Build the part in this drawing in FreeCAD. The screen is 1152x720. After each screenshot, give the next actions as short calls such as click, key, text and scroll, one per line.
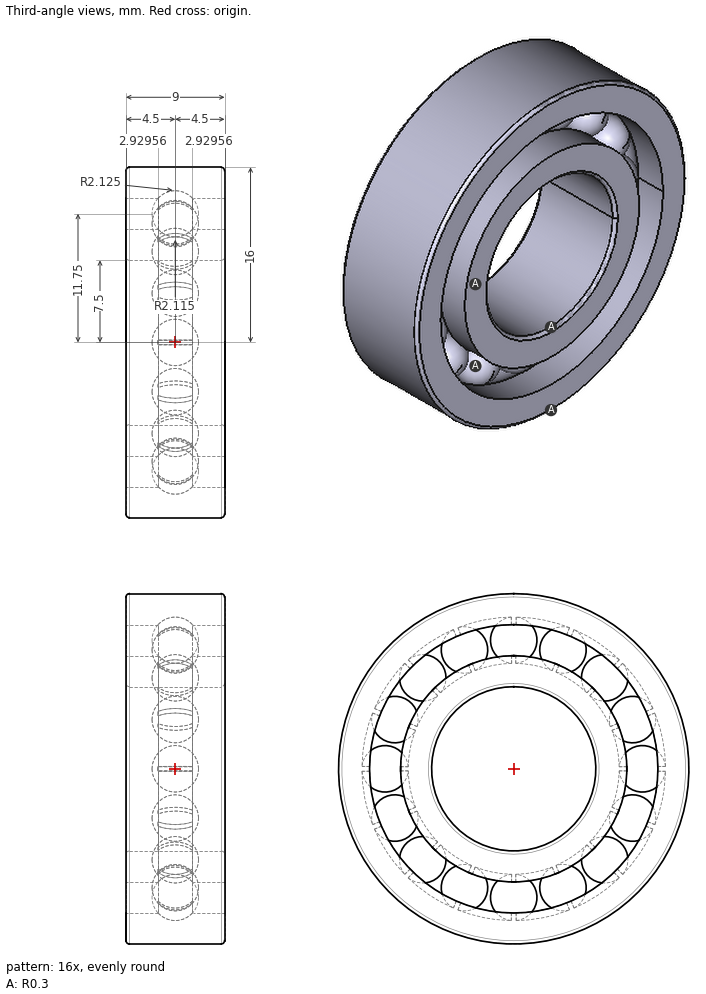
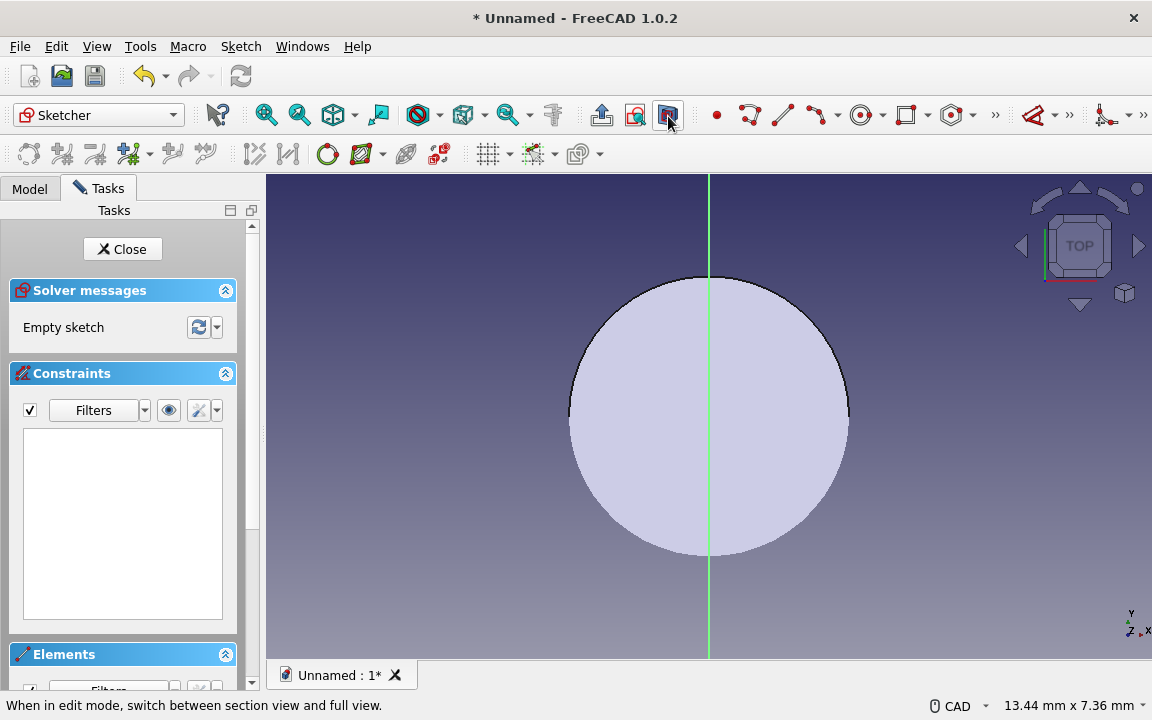
scroll(601, 202, down, 5)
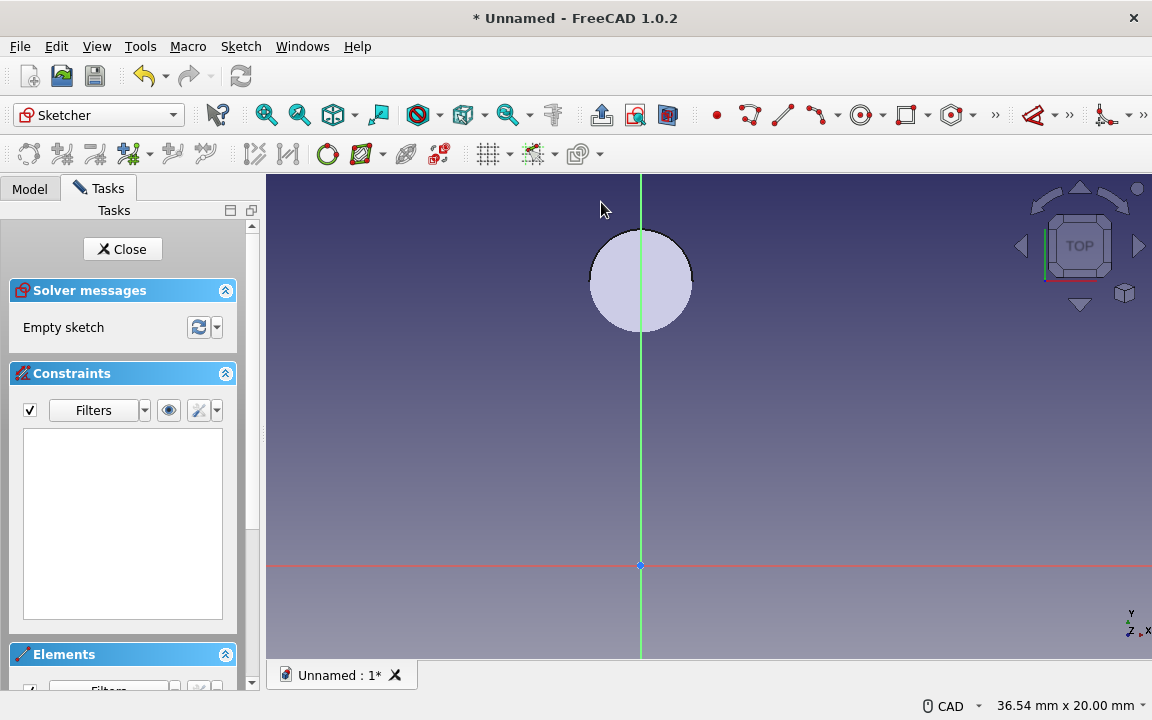
click(750, 116)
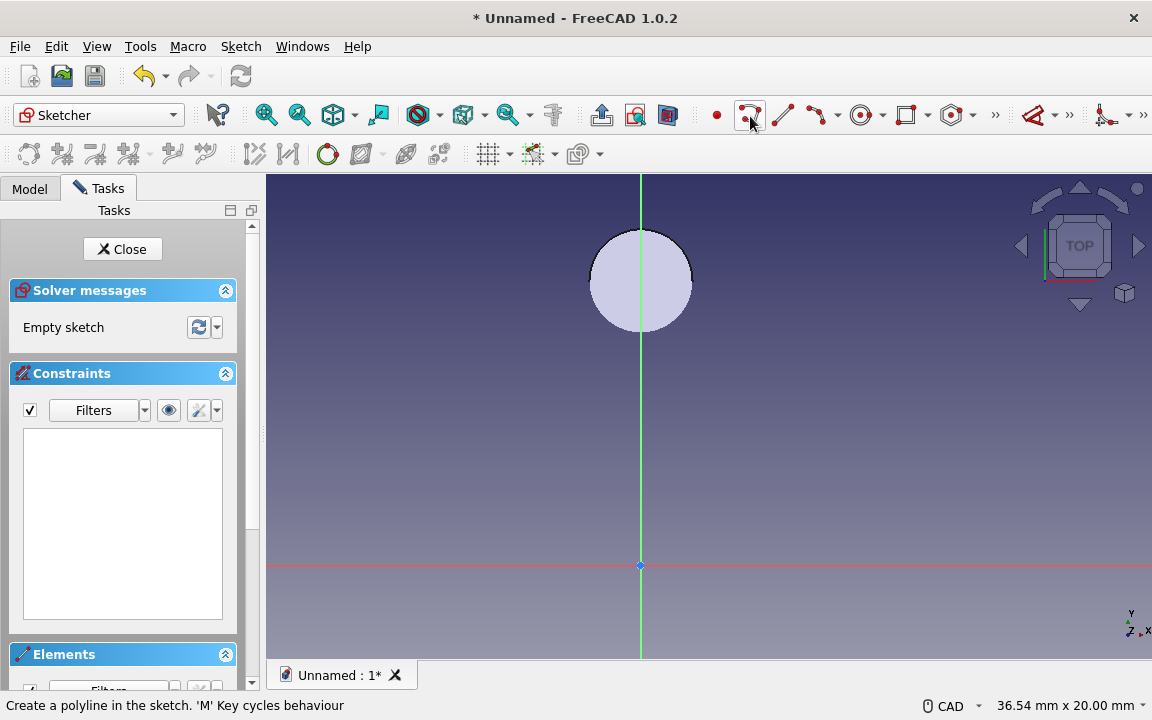
click(603, 315)
click(532, 315)
click(532, 384)
click(750, 384)
click(750, 315)
click(679, 315)
right_click(679, 315)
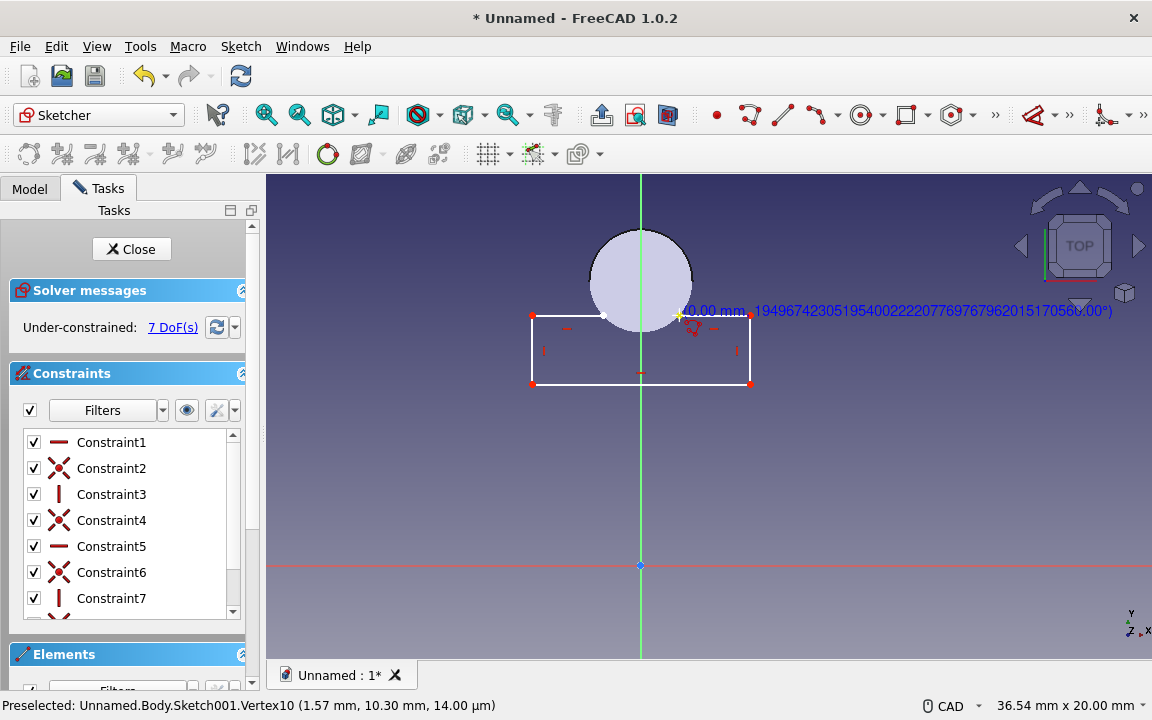
click(816, 116)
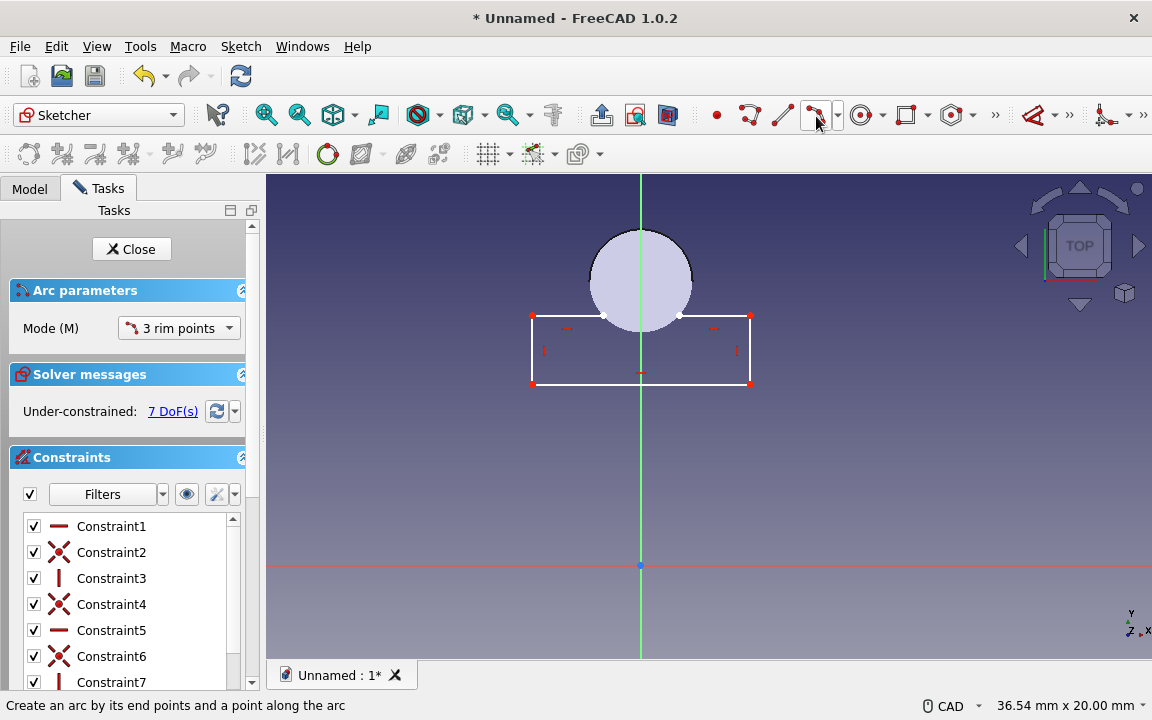
click(679, 316)
click(603, 316)
click(624, 329)
key(Escape)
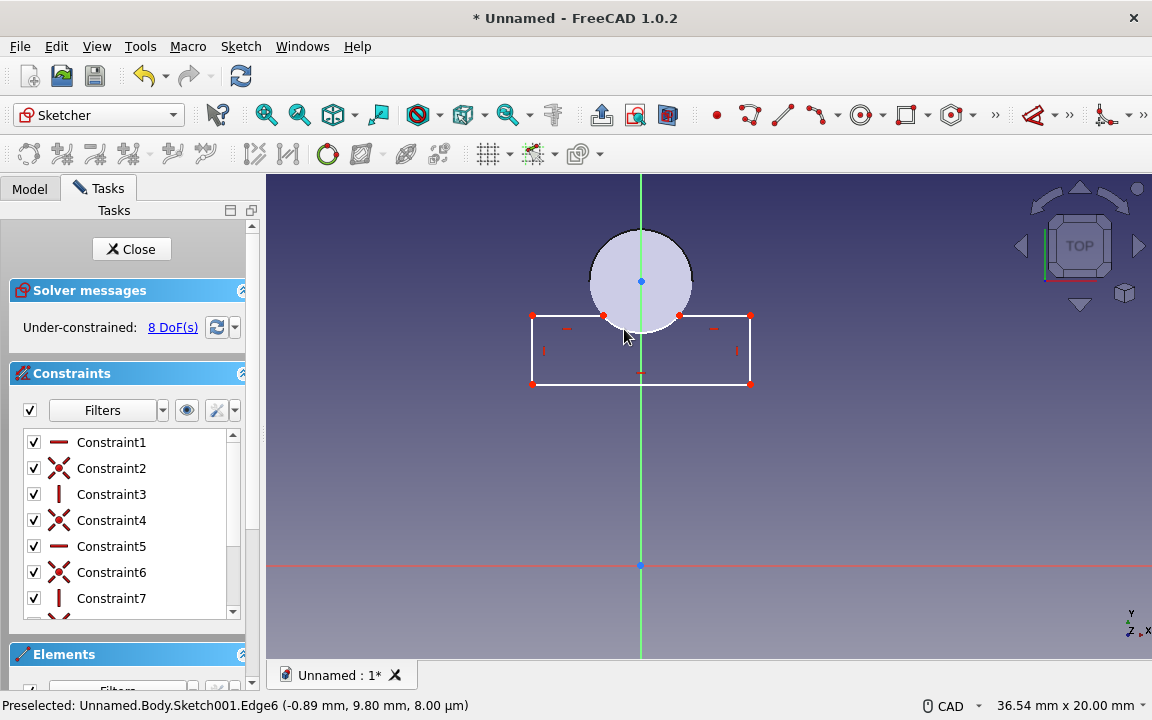
click(641, 282)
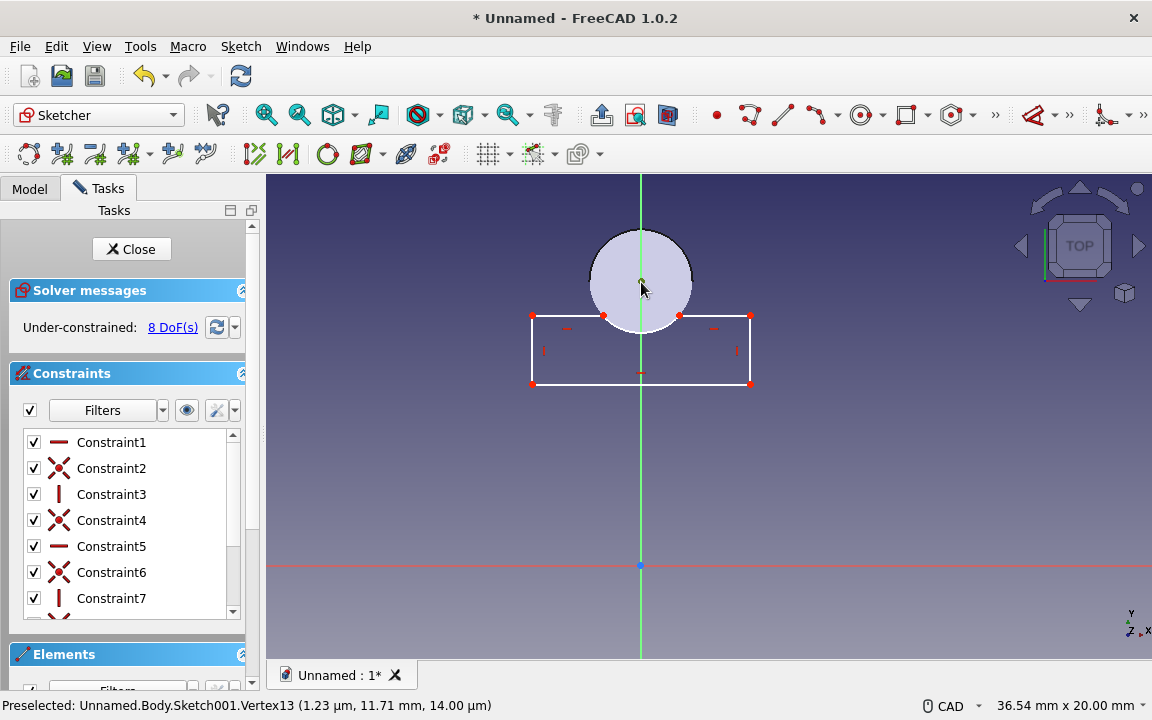
click(641, 600)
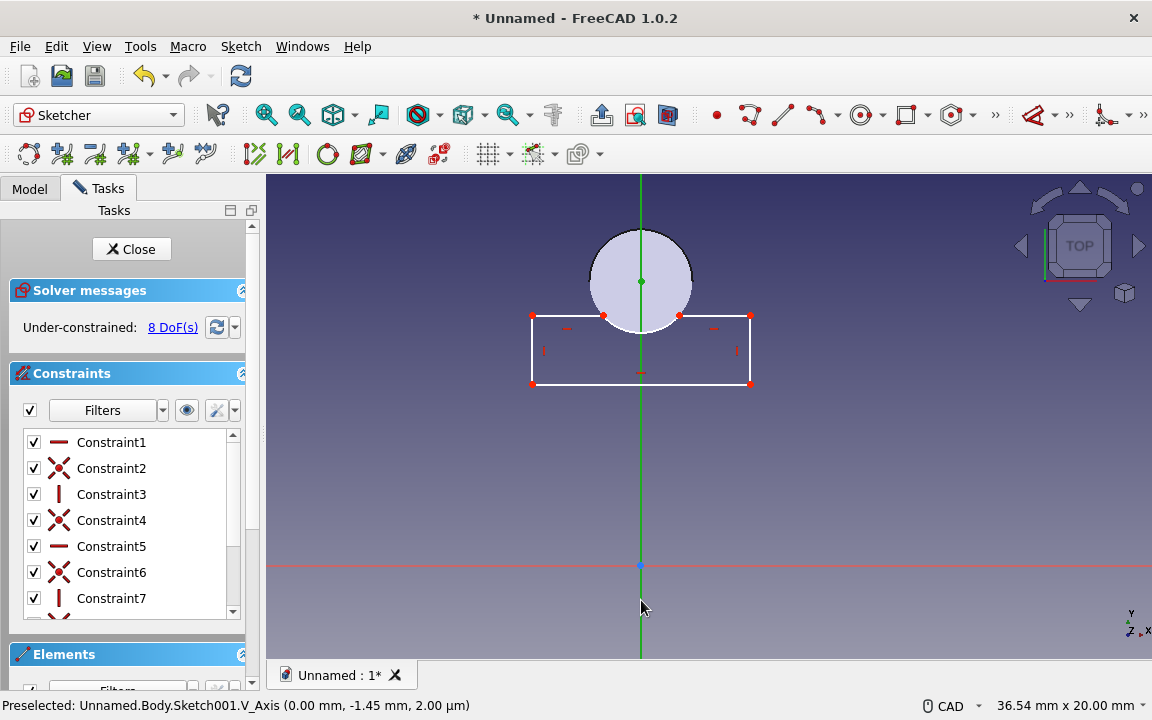
key(c)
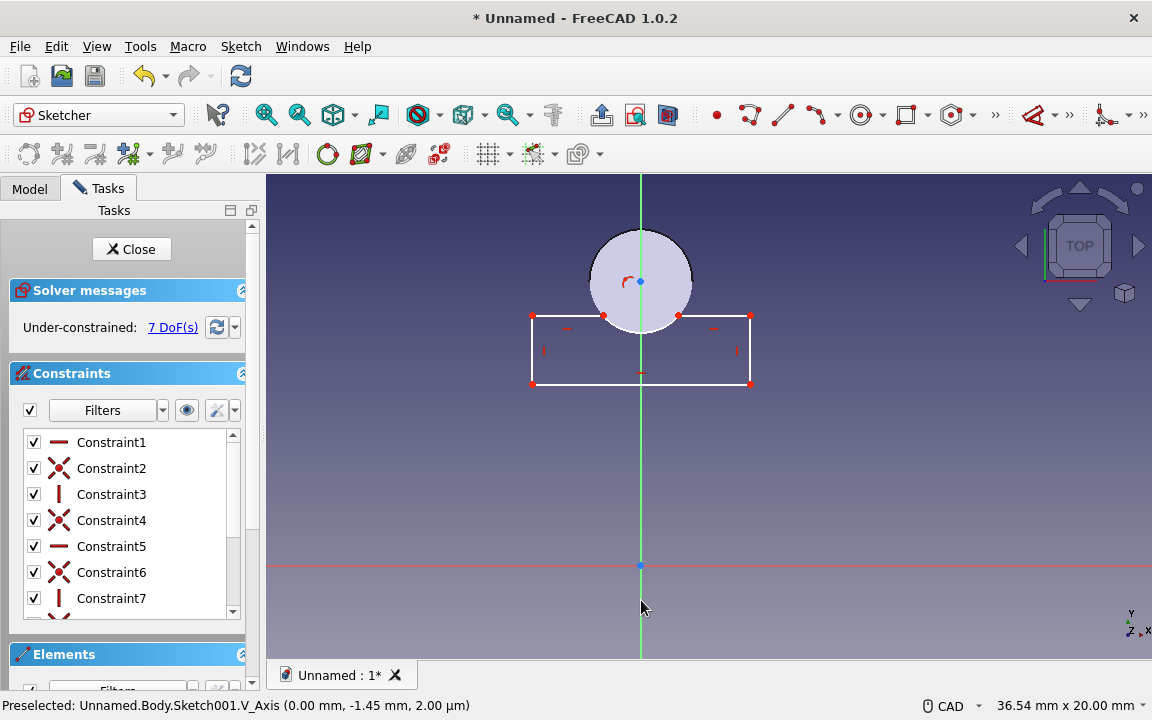
click(1032, 116)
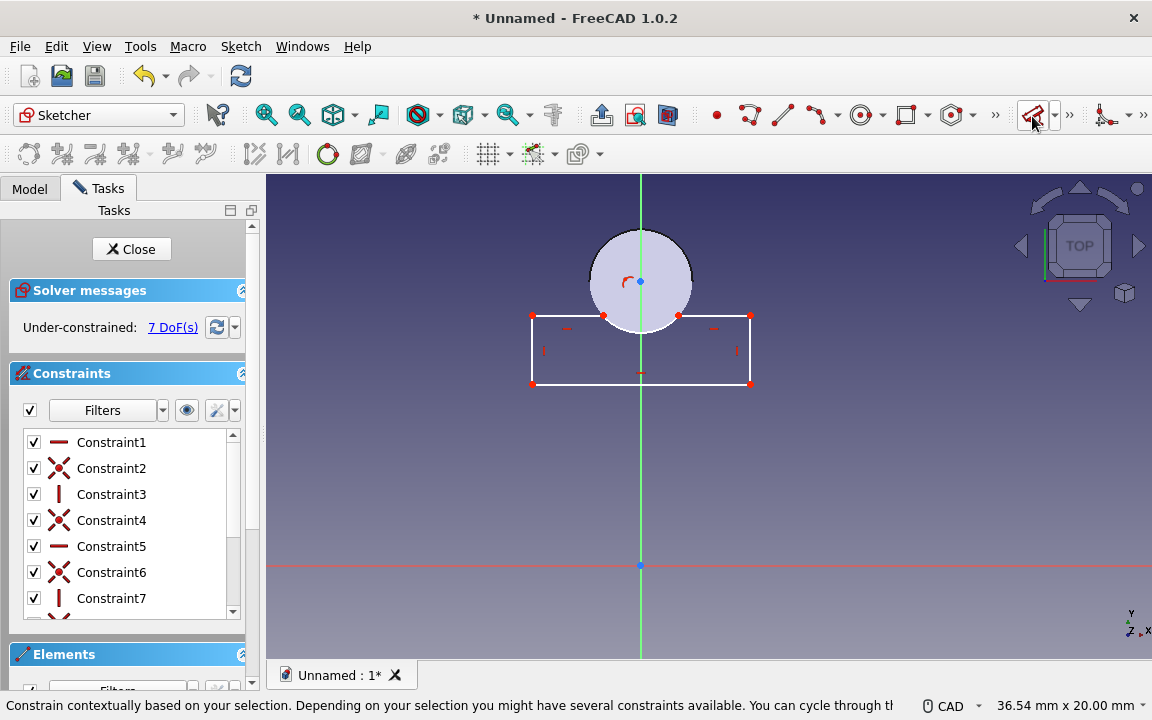
click(624, 330)
click(613, 360)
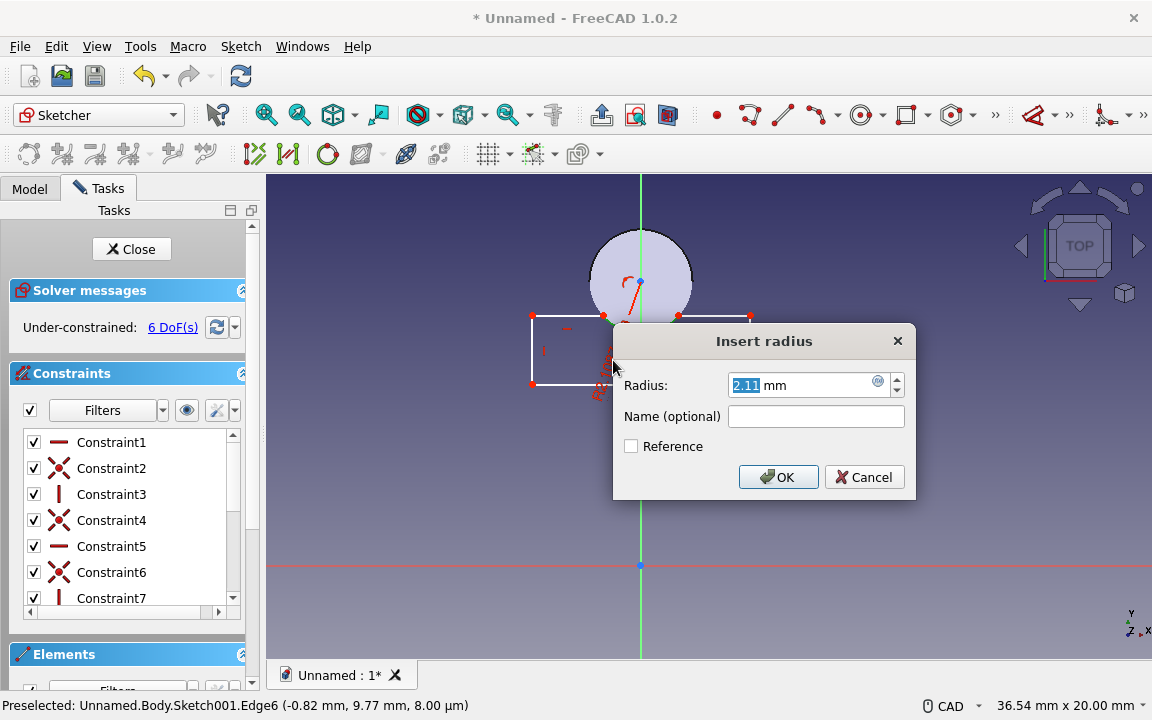
text(2.115)
key(Return)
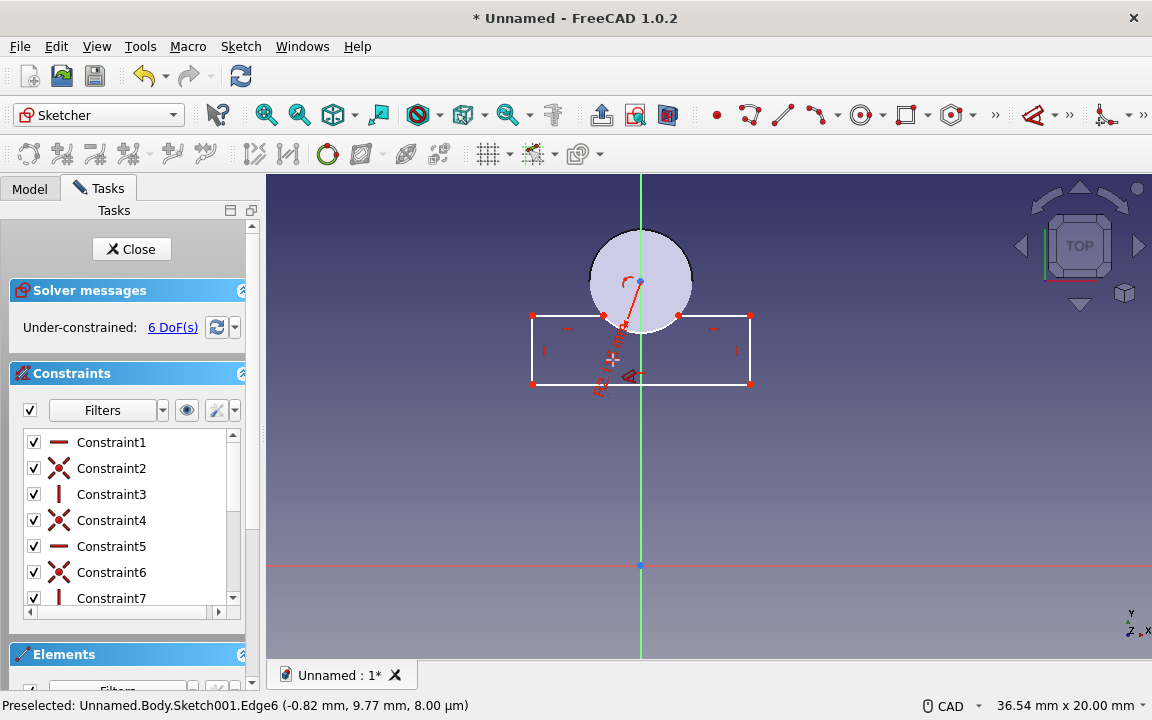
click(597, 385)
click(691, 351)